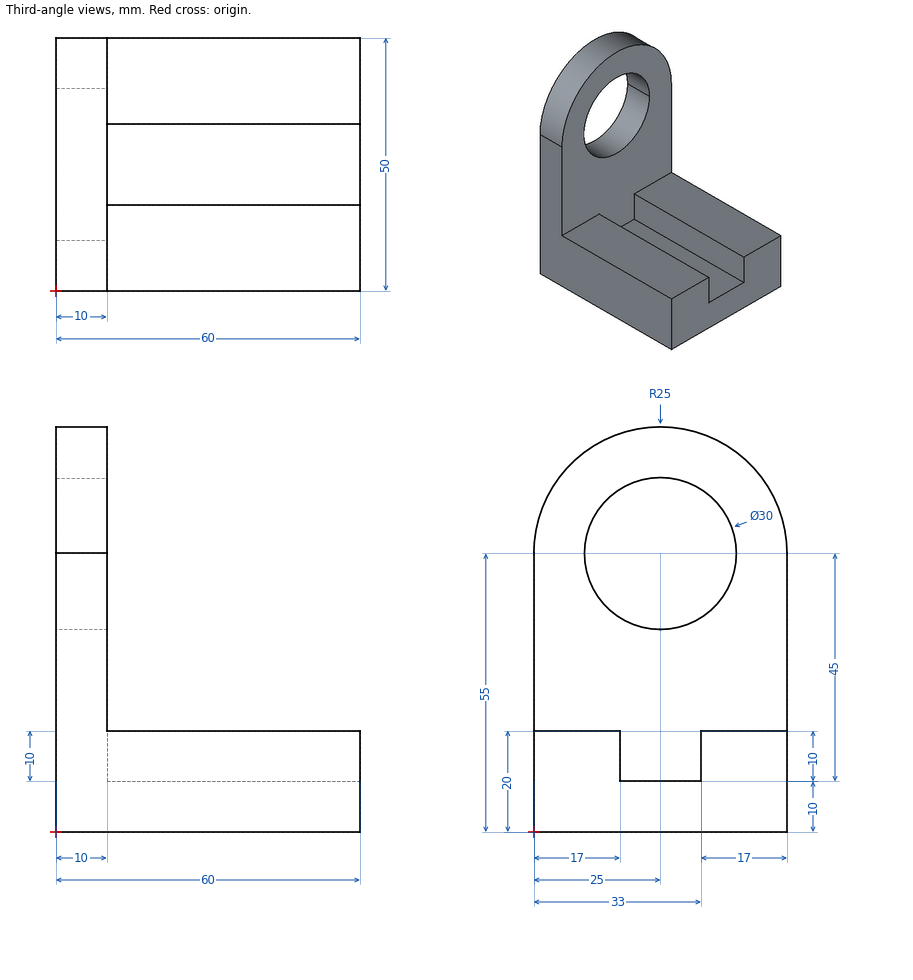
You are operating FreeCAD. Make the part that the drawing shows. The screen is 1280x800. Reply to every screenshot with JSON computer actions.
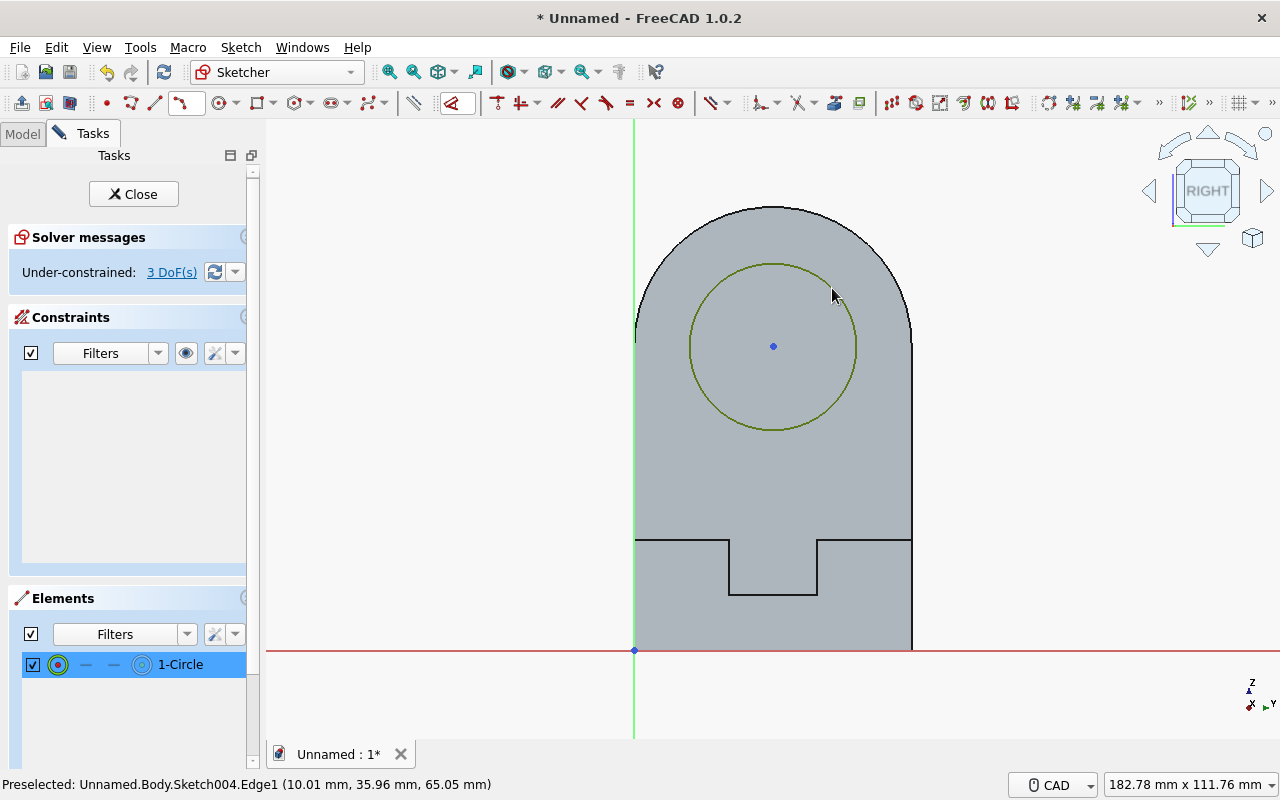
{"action": "left_click", "coordinate": [470, 104]}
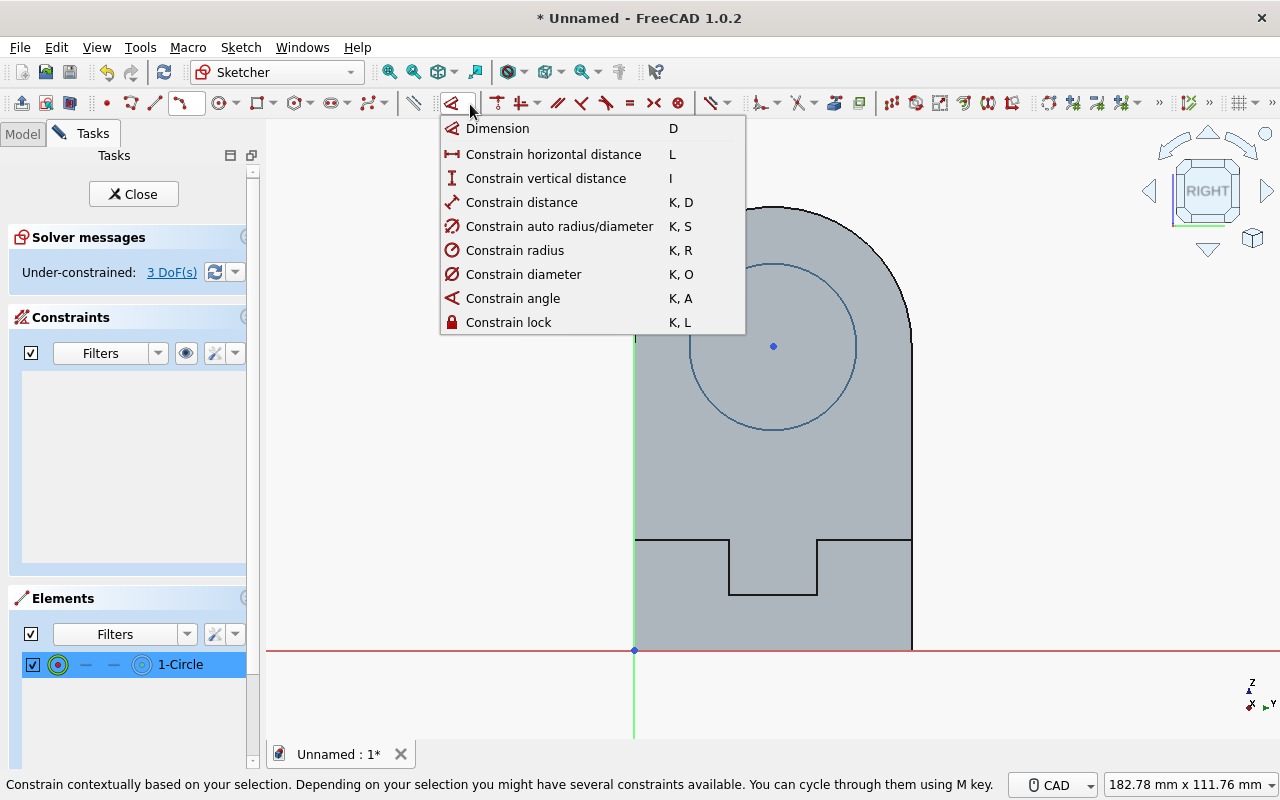
{"action": "left_click", "coordinate": [593, 274]}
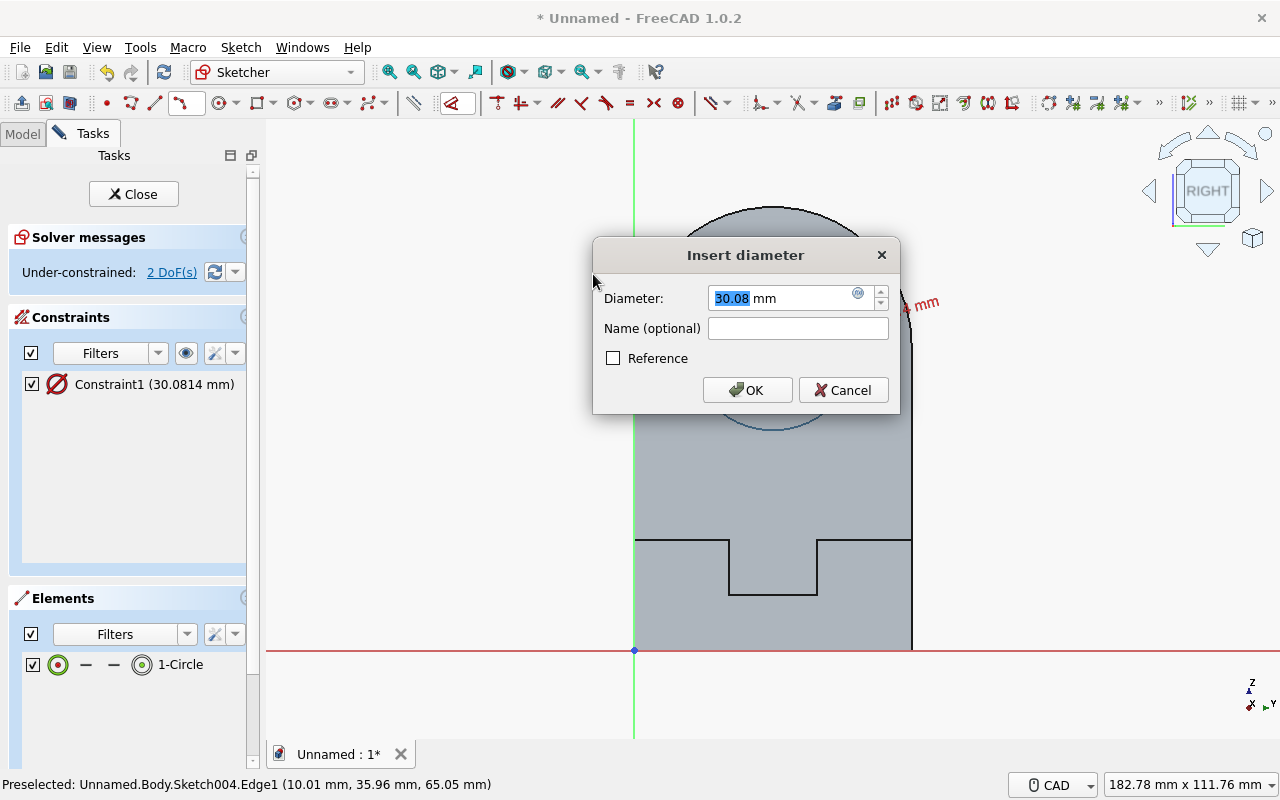
{"action": "type", "text": "30"}
{"action": "key", "text": "Return"}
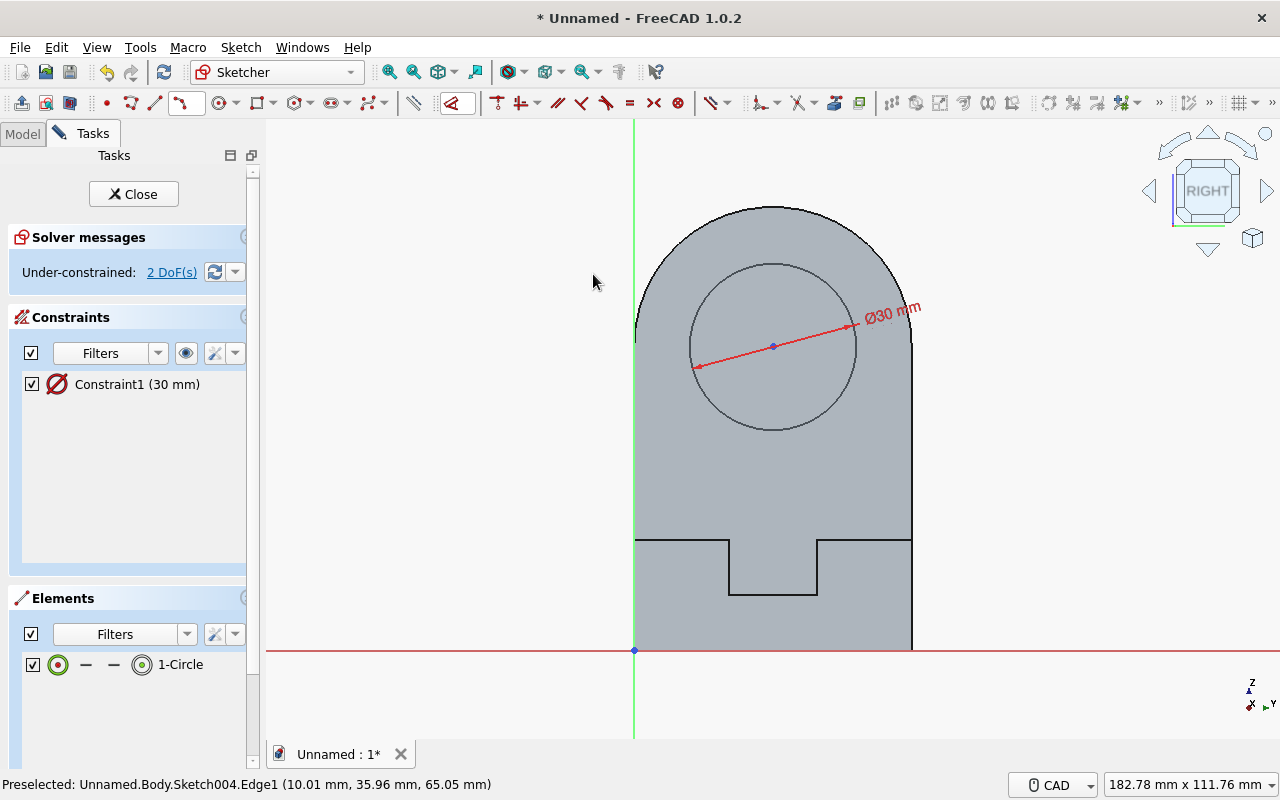
{"action": "left_click", "coordinate": [773, 347]}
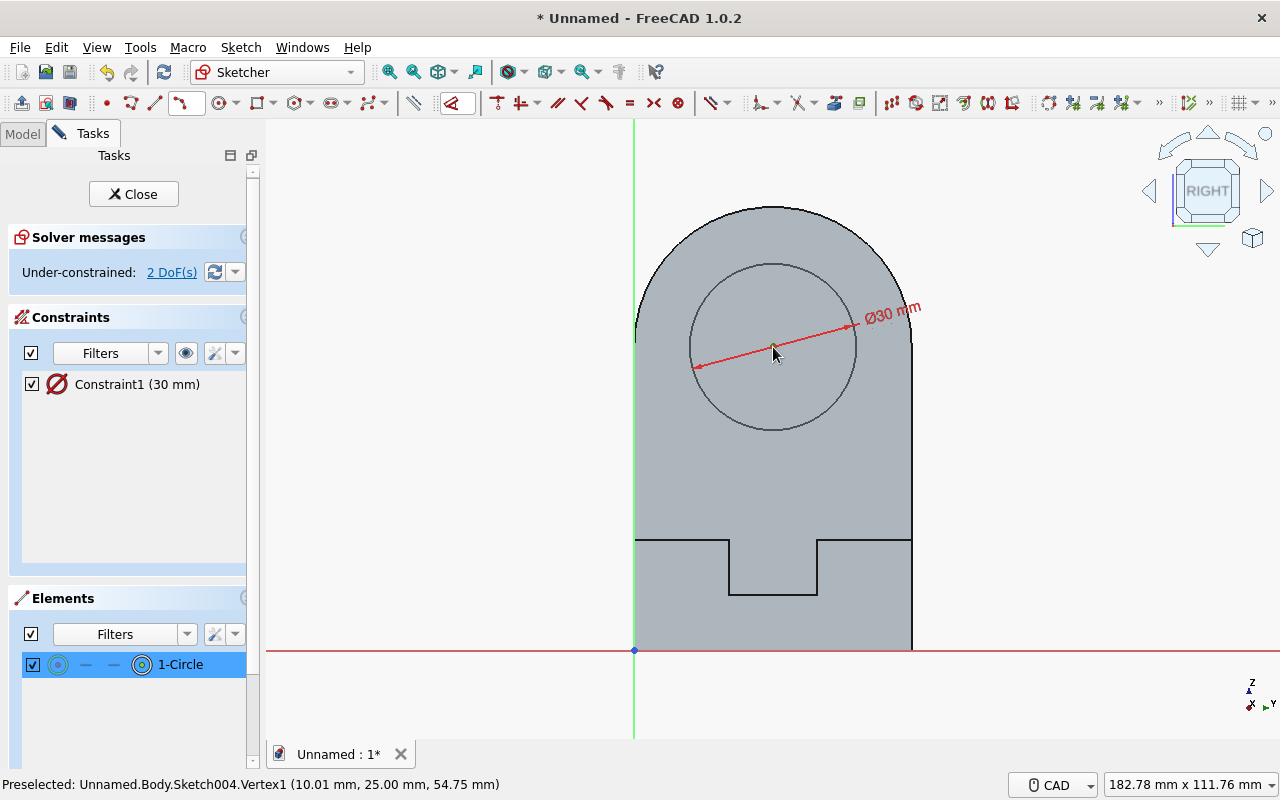
{"action": "left_click", "coordinate": [470, 104]}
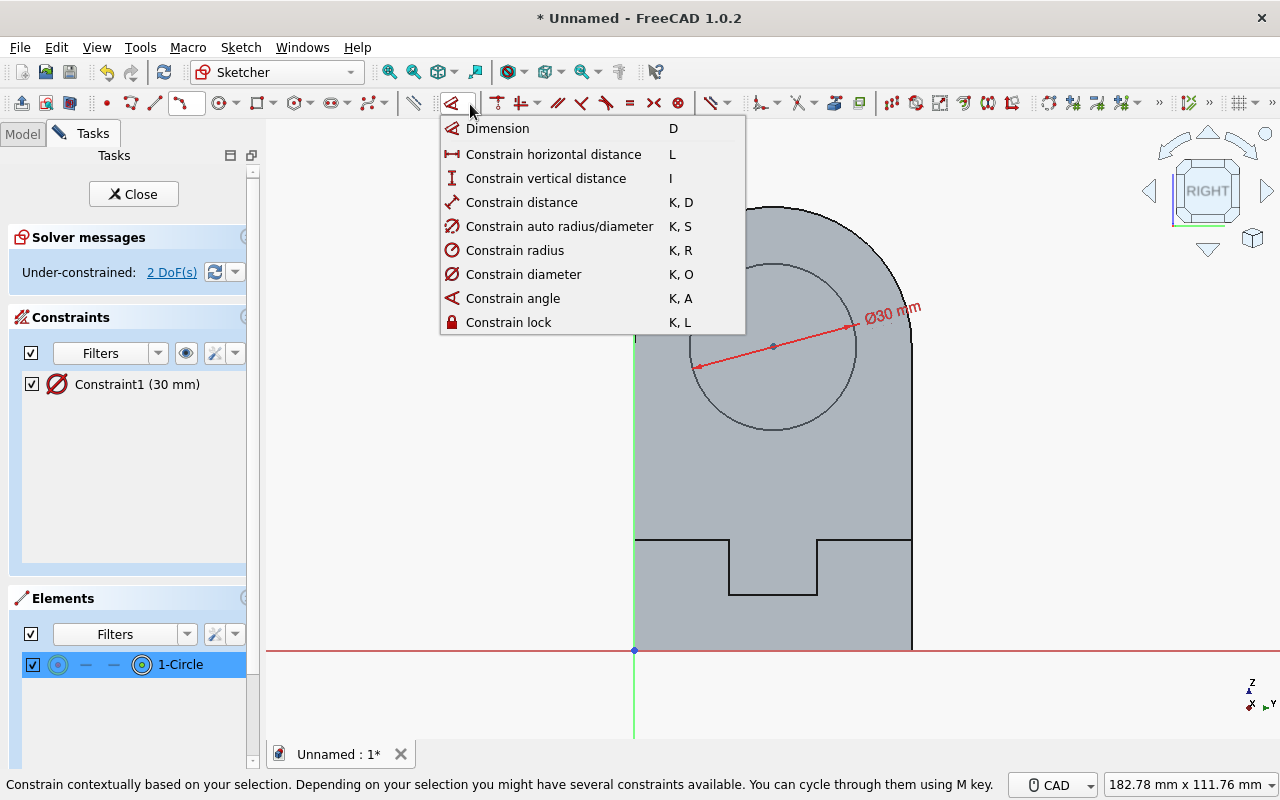
{"action": "left_click", "coordinate": [593, 154]}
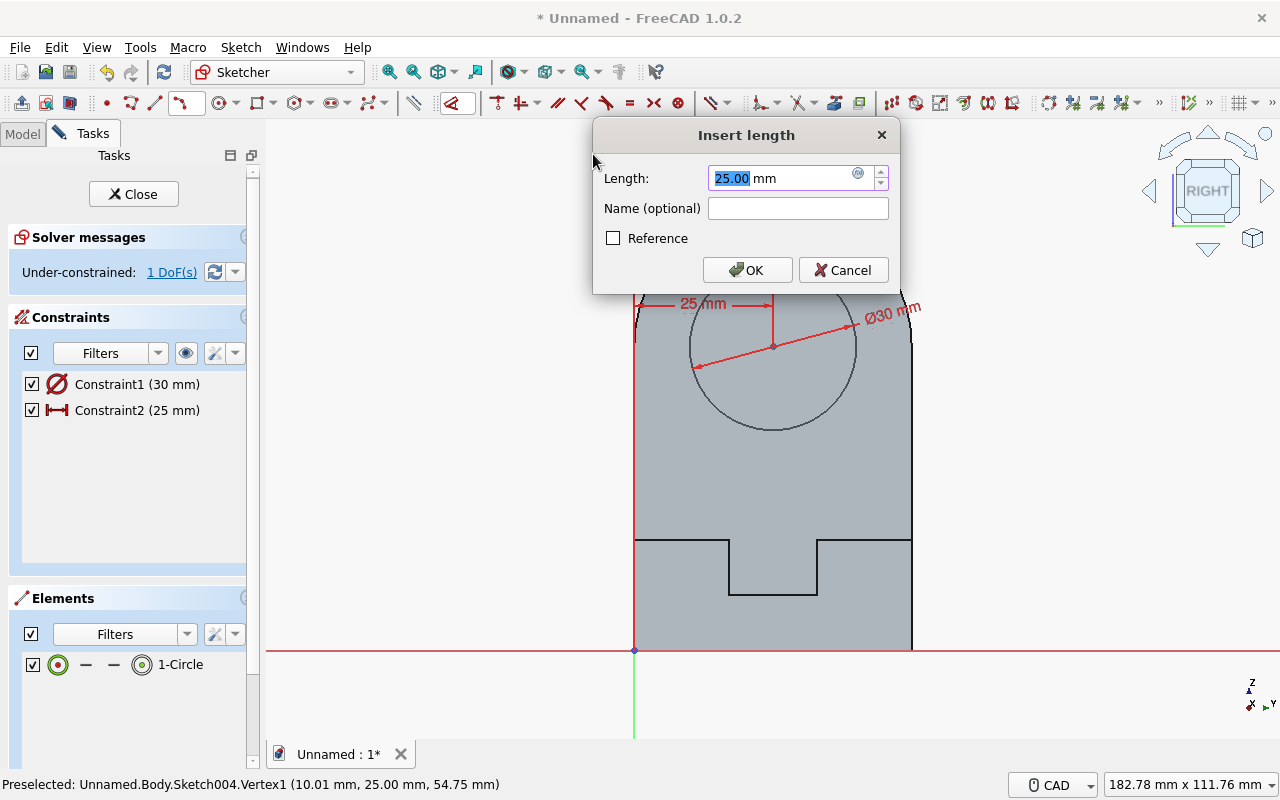
{"action": "type", "text": "25"}
{"action": "key", "text": "Return"}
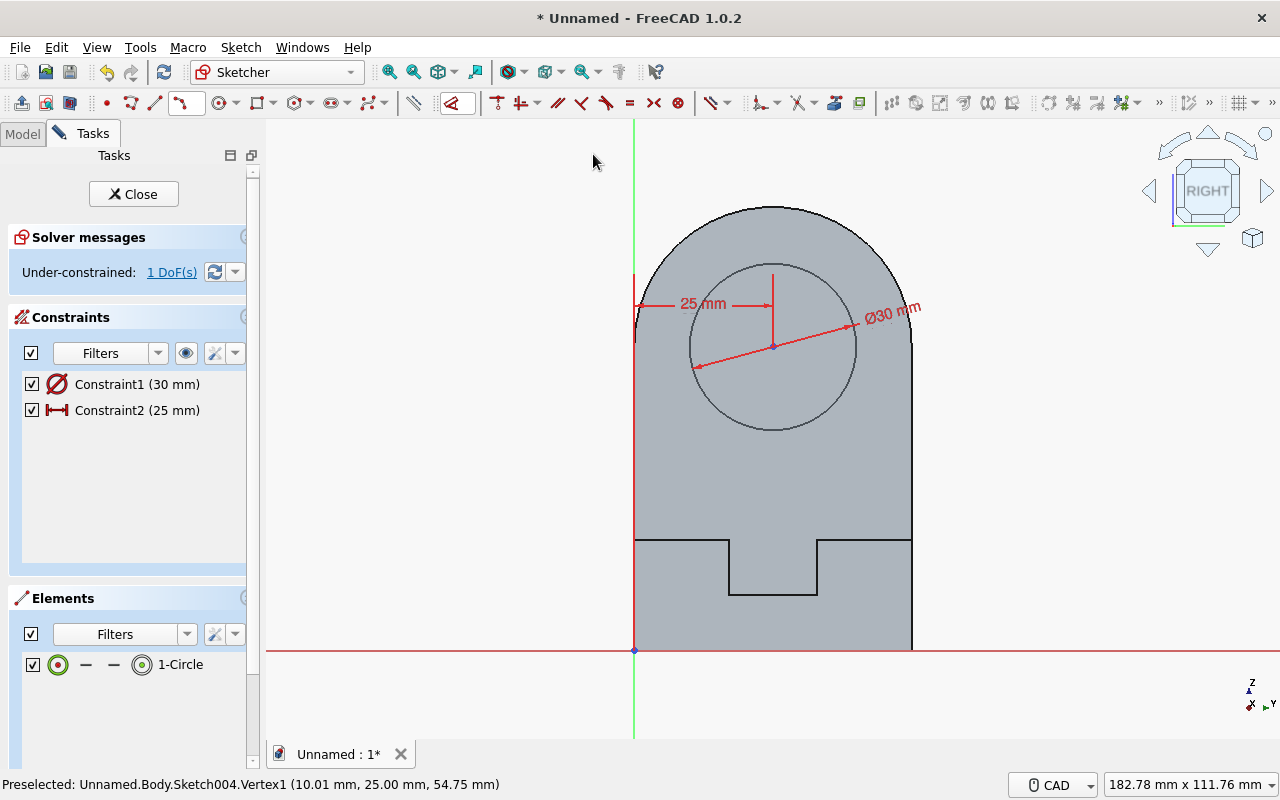
{"action": "left_click", "coordinate": [773, 347]}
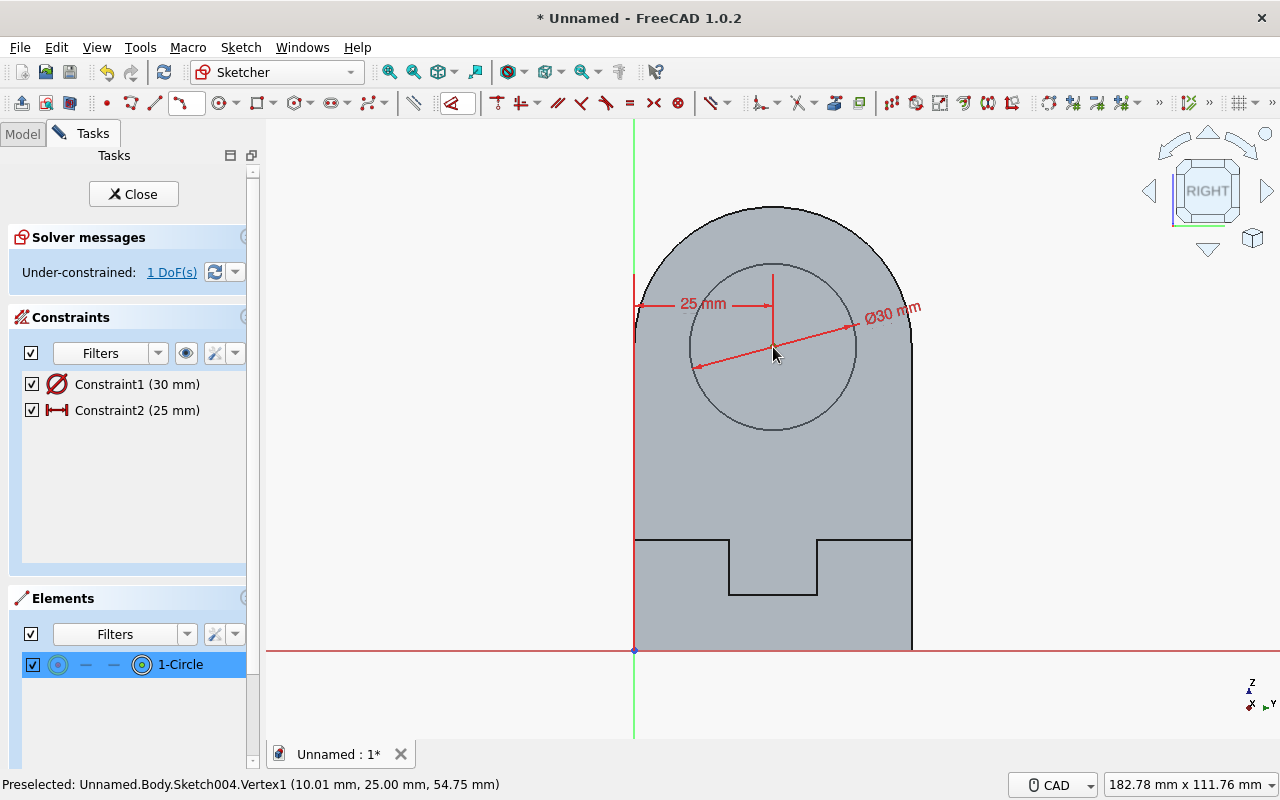
{"action": "key", "text": "i"}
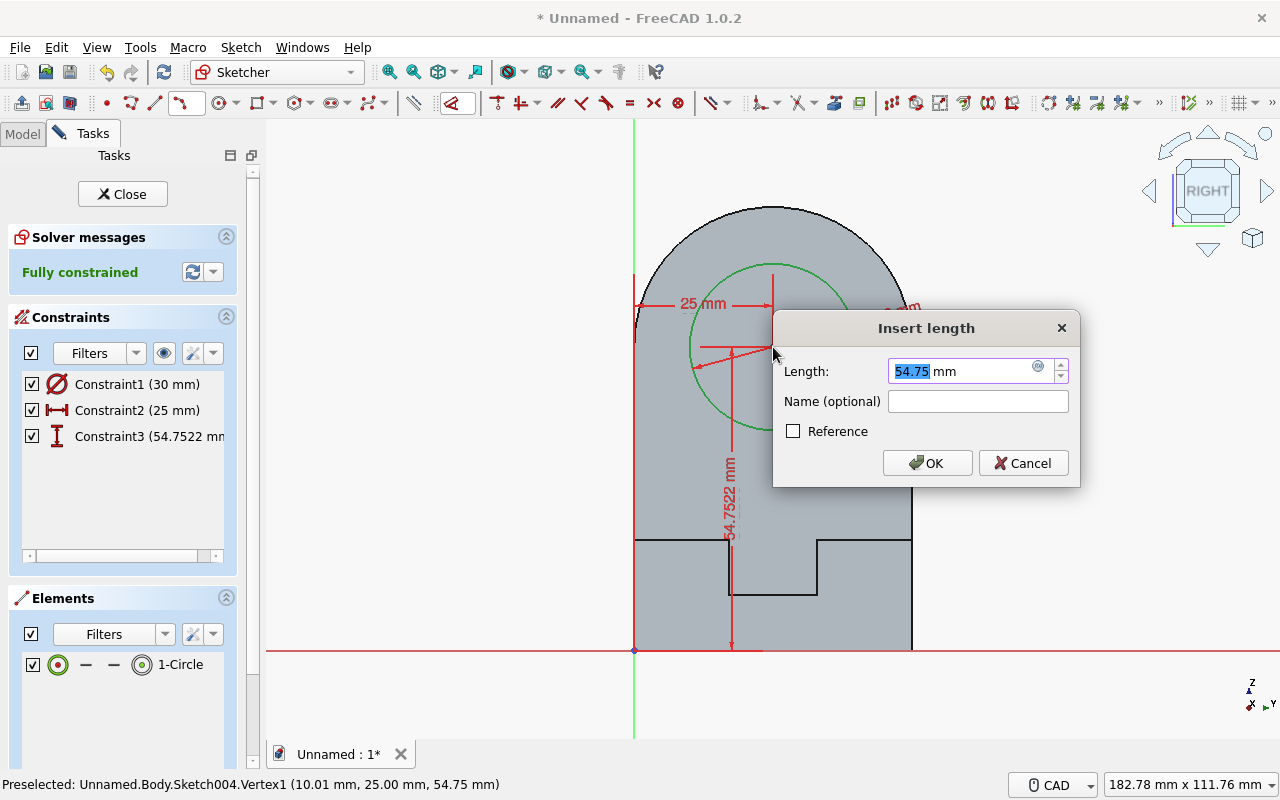
{"action": "type", "text": "55"}
{"action": "key", "text": "Return"}